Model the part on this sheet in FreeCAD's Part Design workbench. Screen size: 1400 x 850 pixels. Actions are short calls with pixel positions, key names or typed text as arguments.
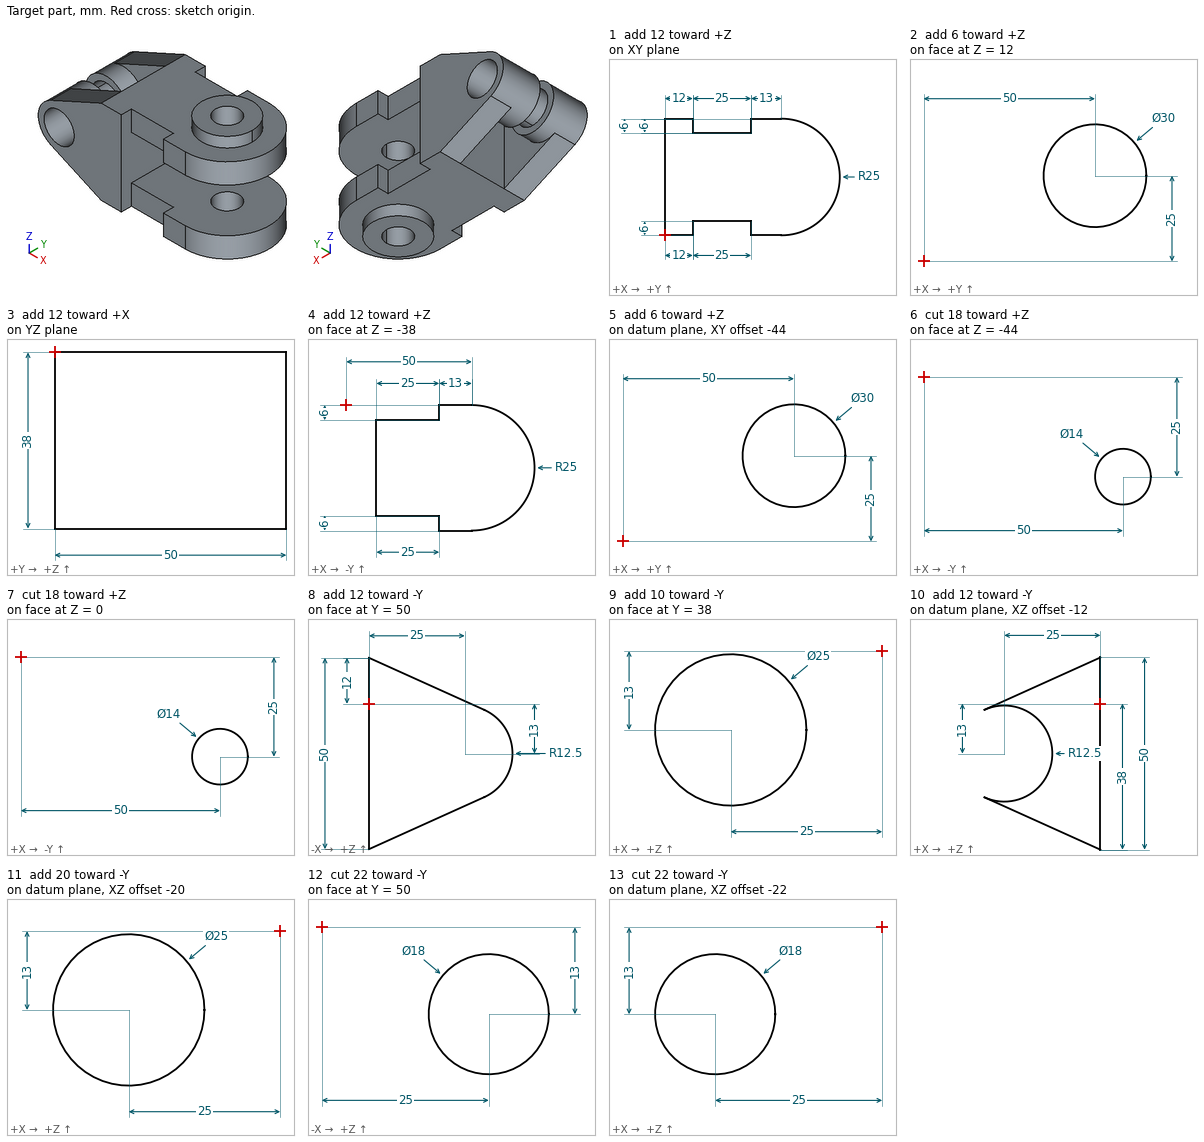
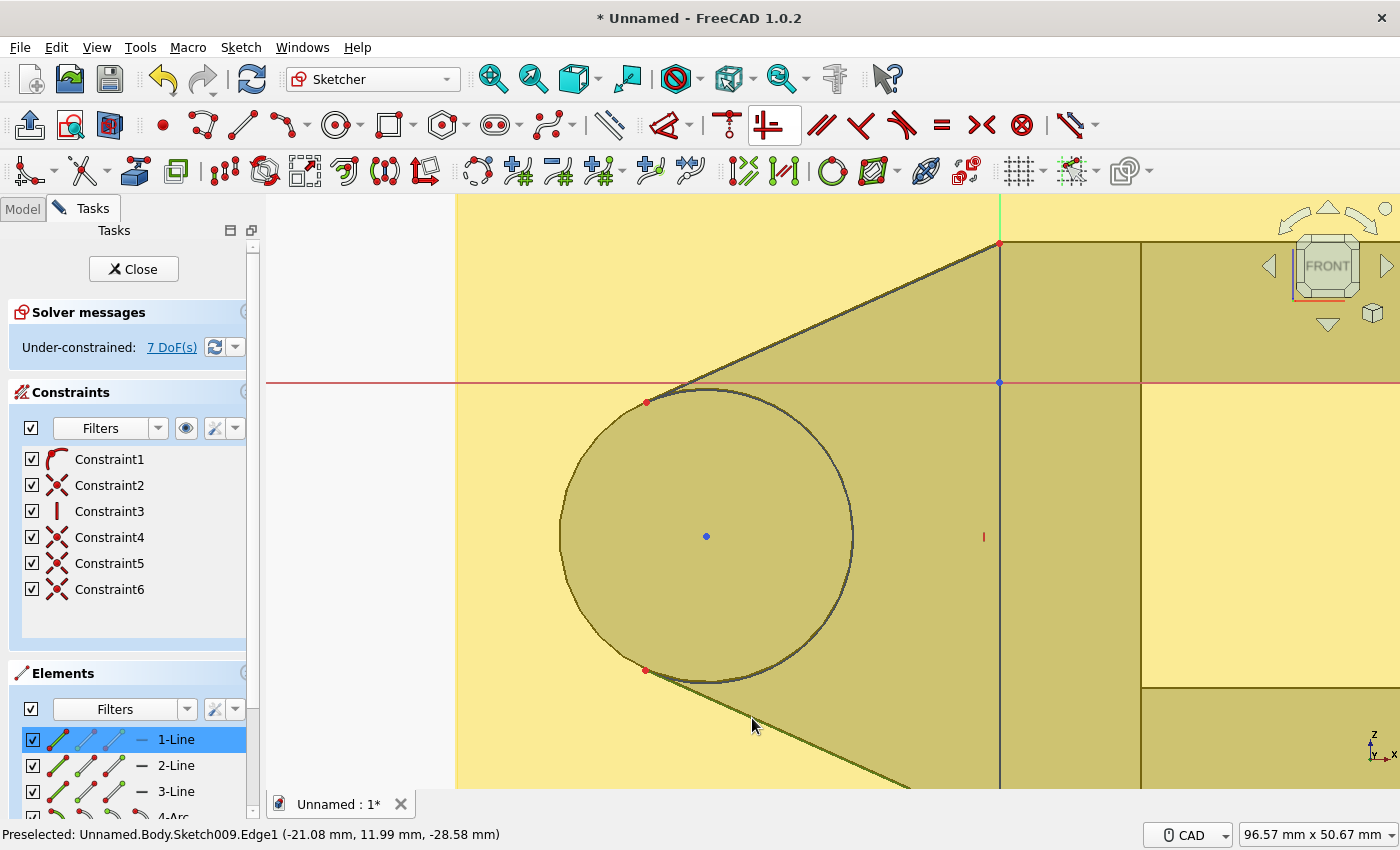
click(809, 642)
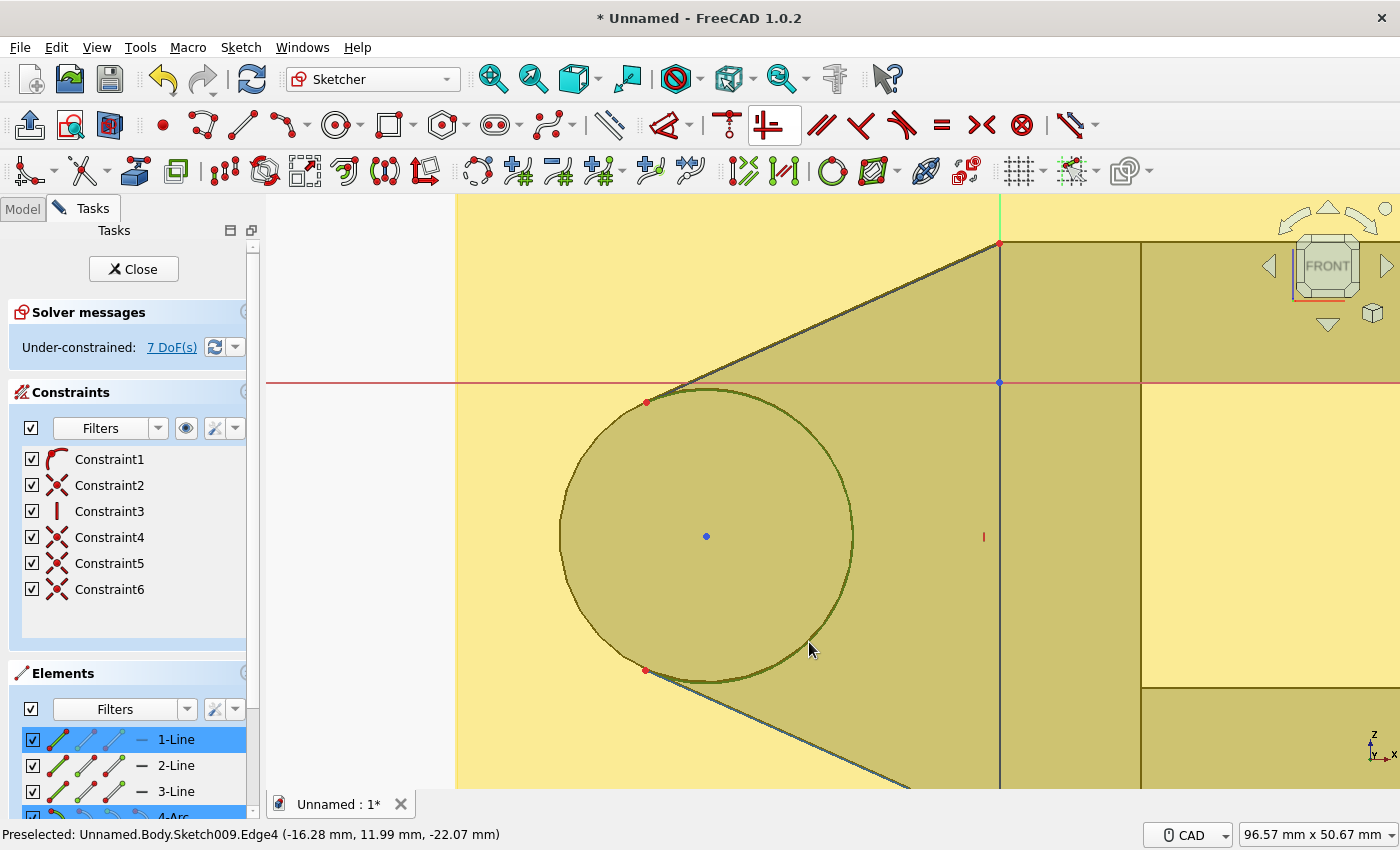
click(902, 126)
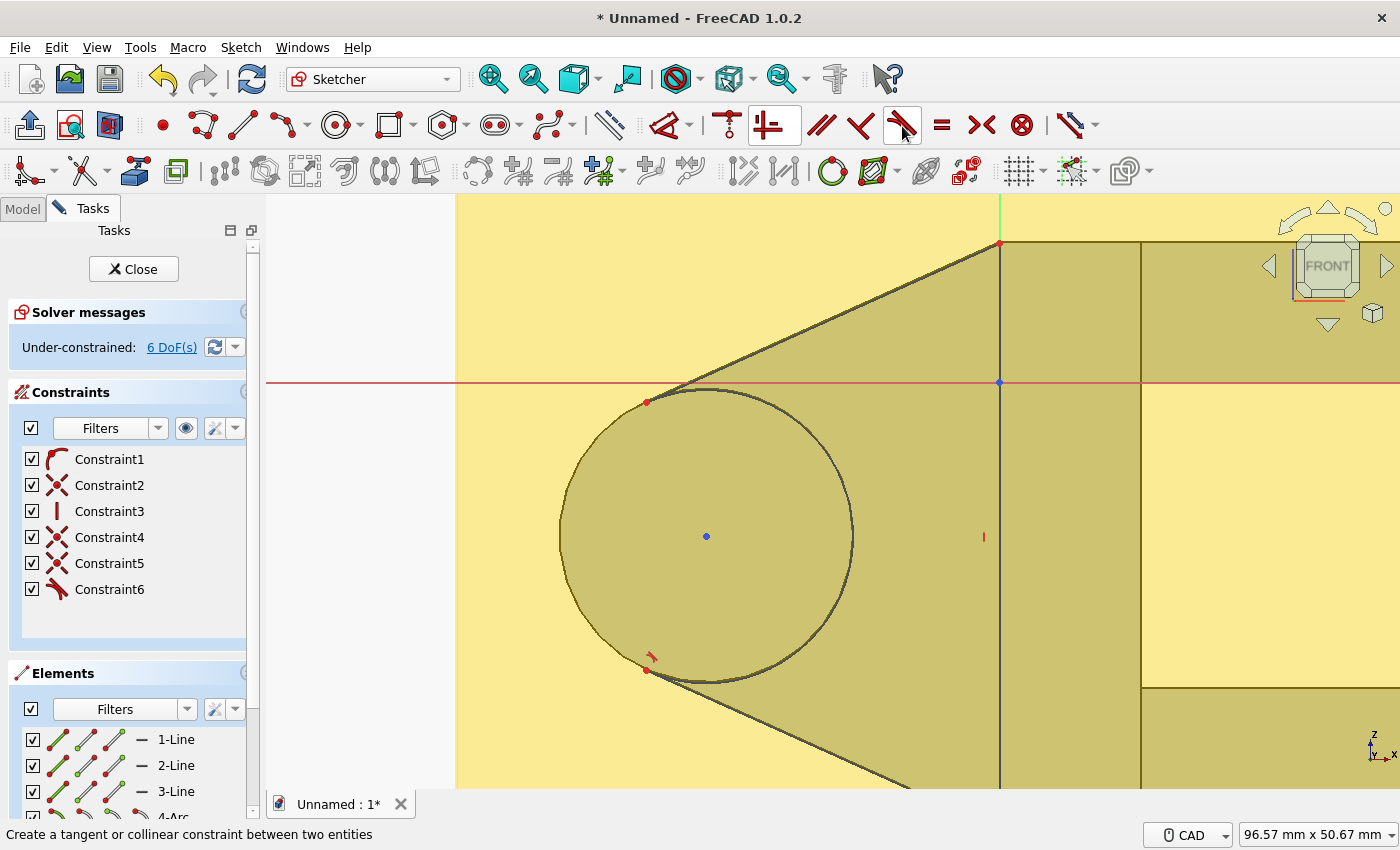
click(894, 291)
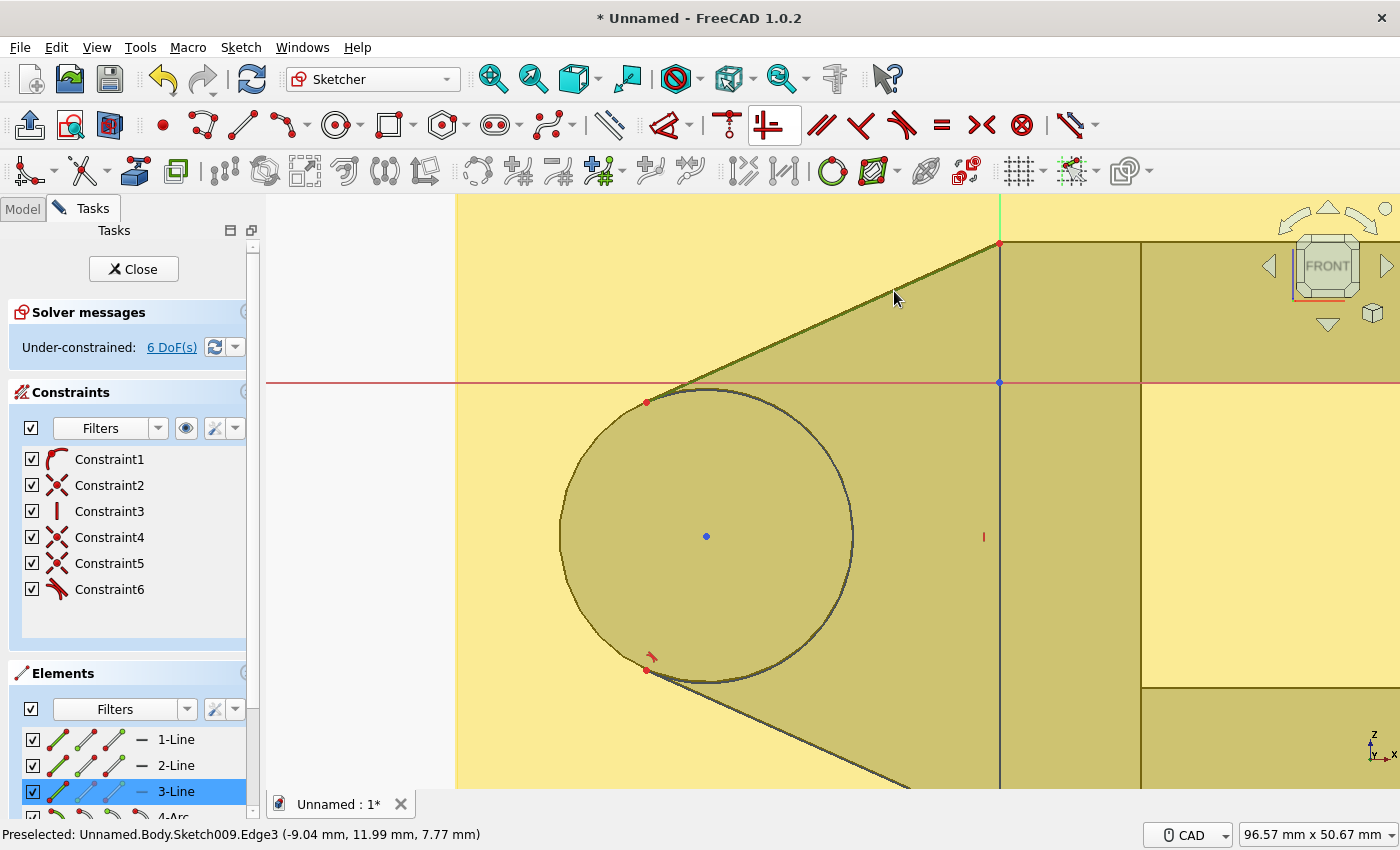
click(809, 642)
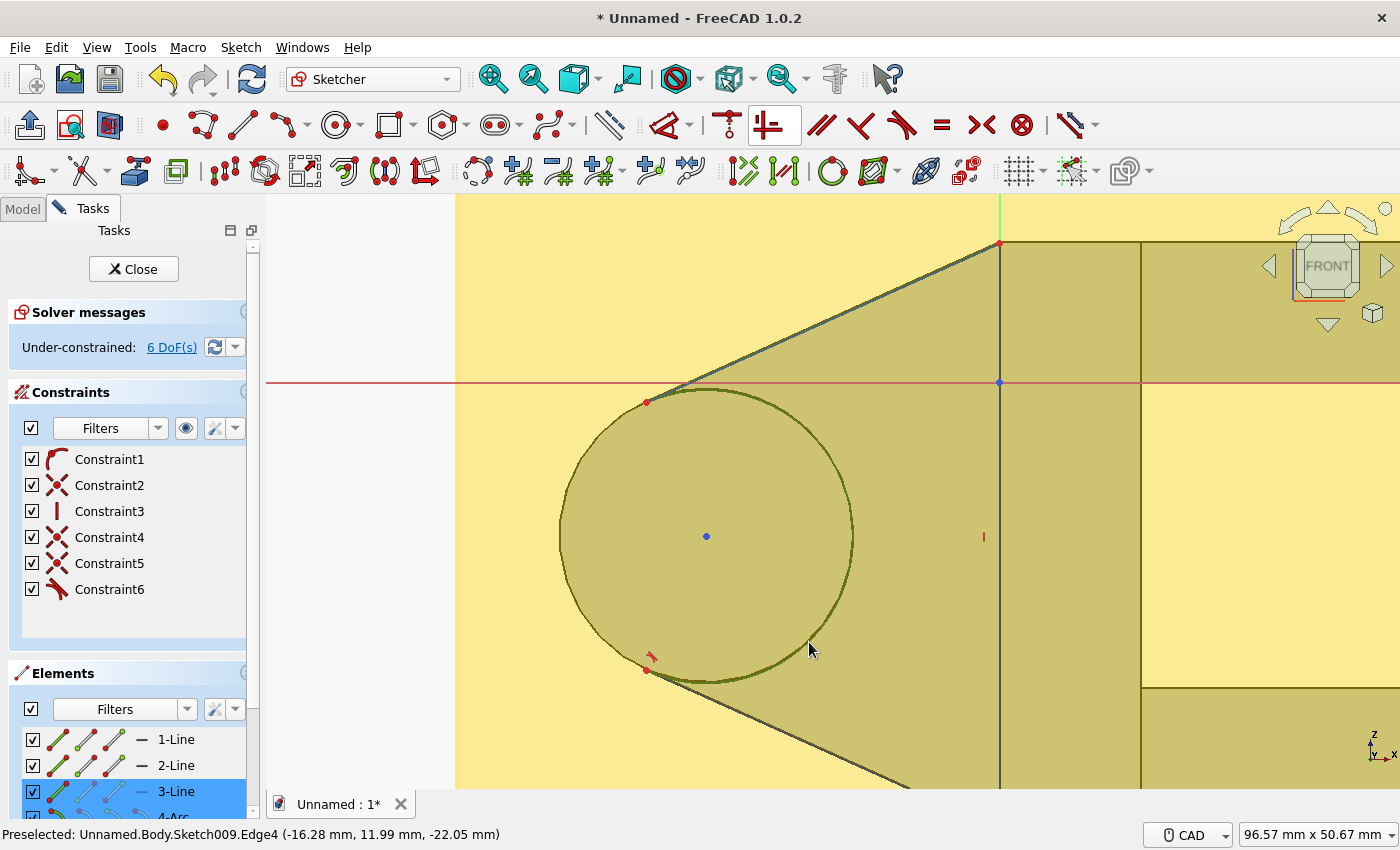
click(902, 126)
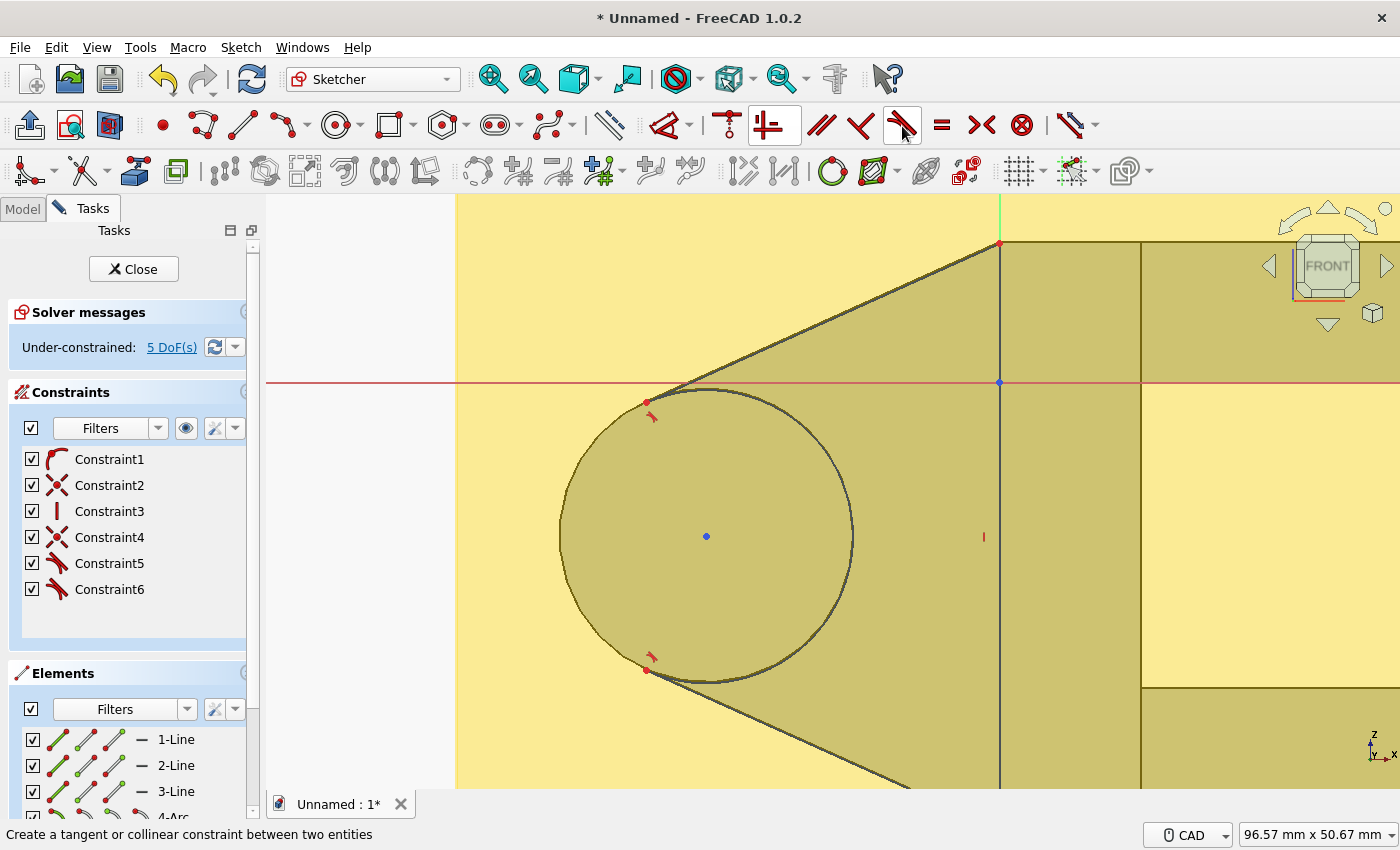
click(664, 126)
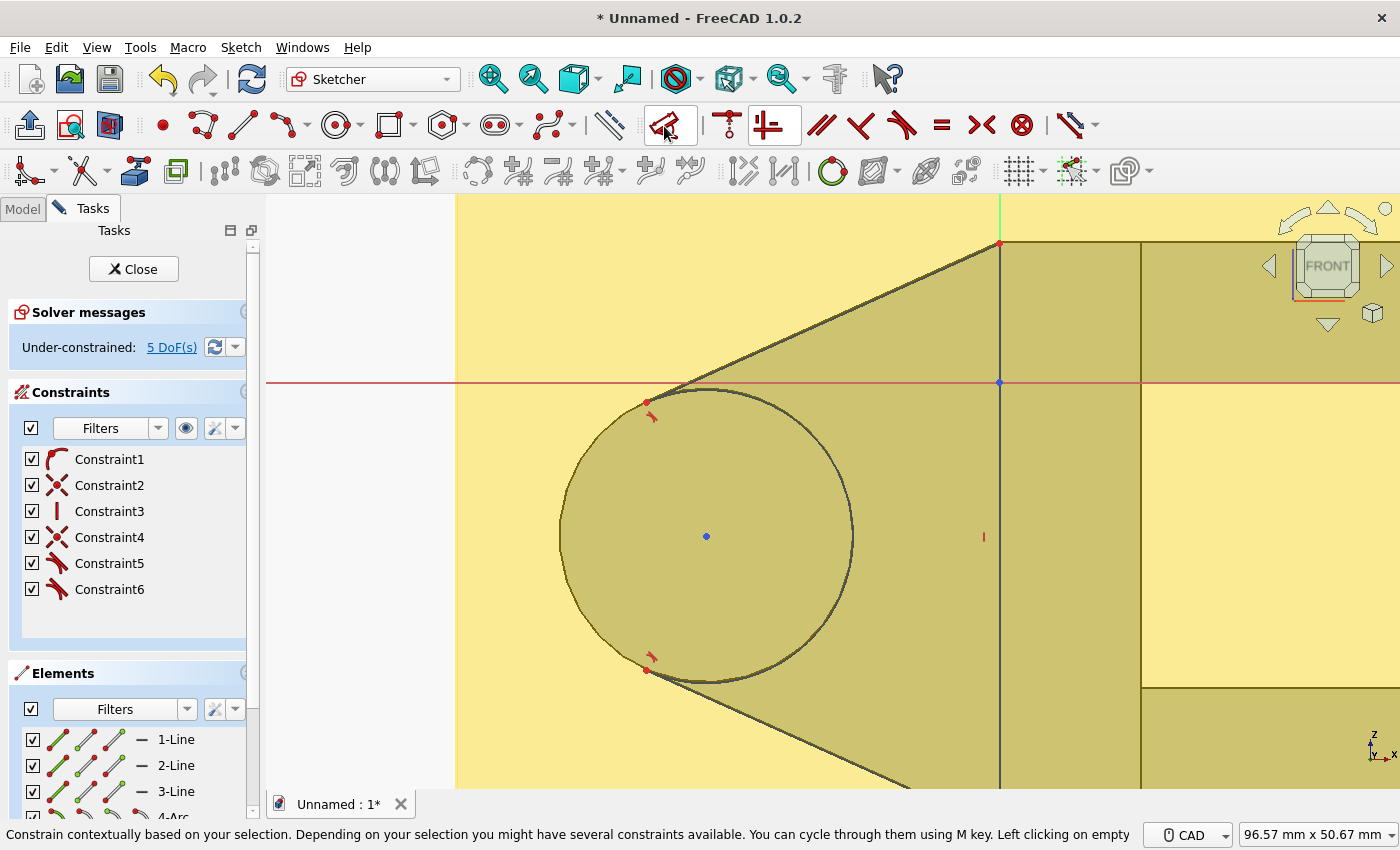
click(809, 642)
click(831, 665)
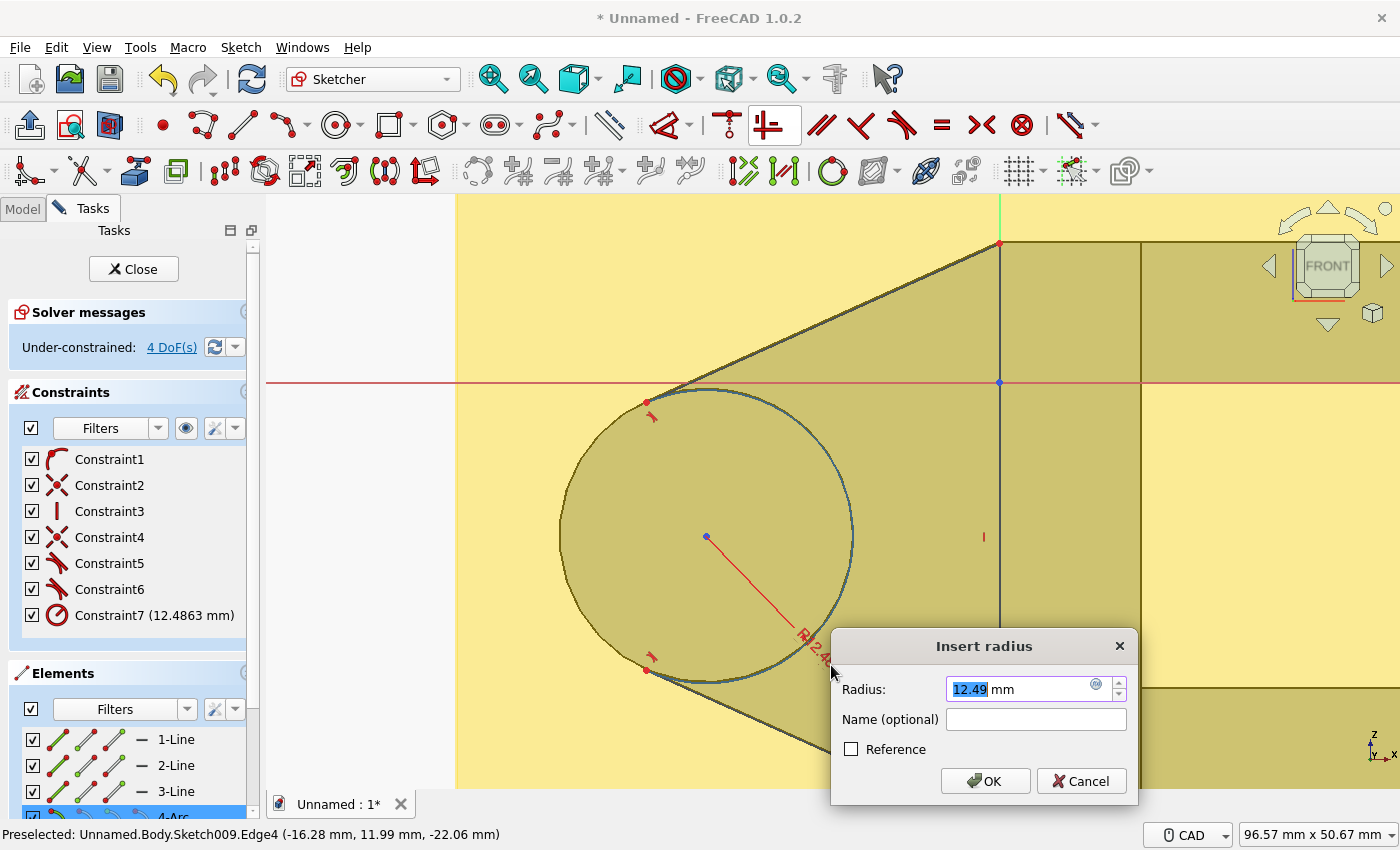
text(12.5)
key(Return)